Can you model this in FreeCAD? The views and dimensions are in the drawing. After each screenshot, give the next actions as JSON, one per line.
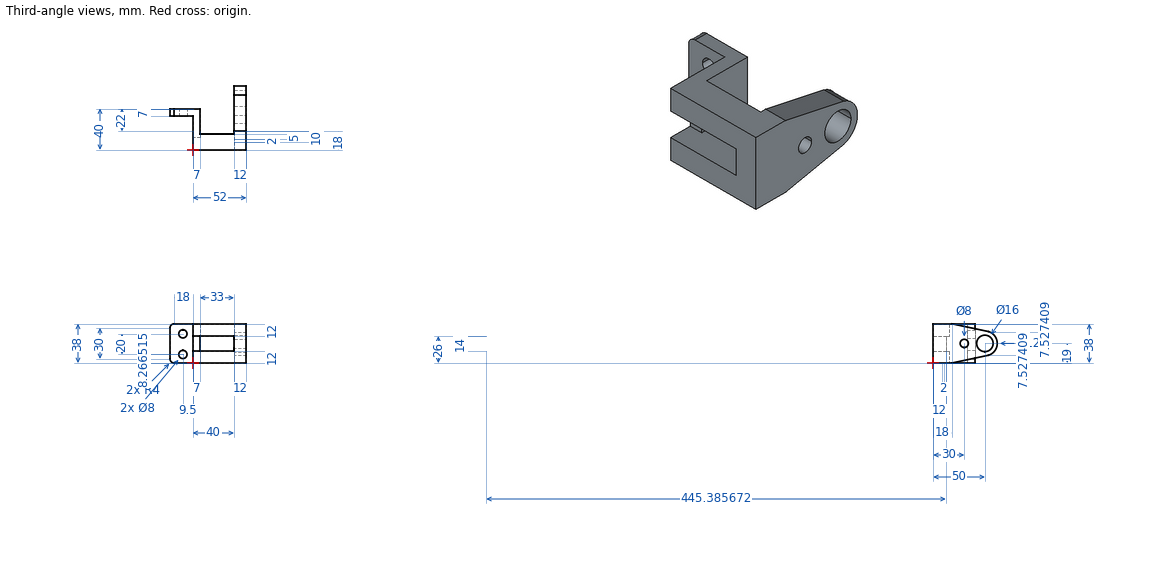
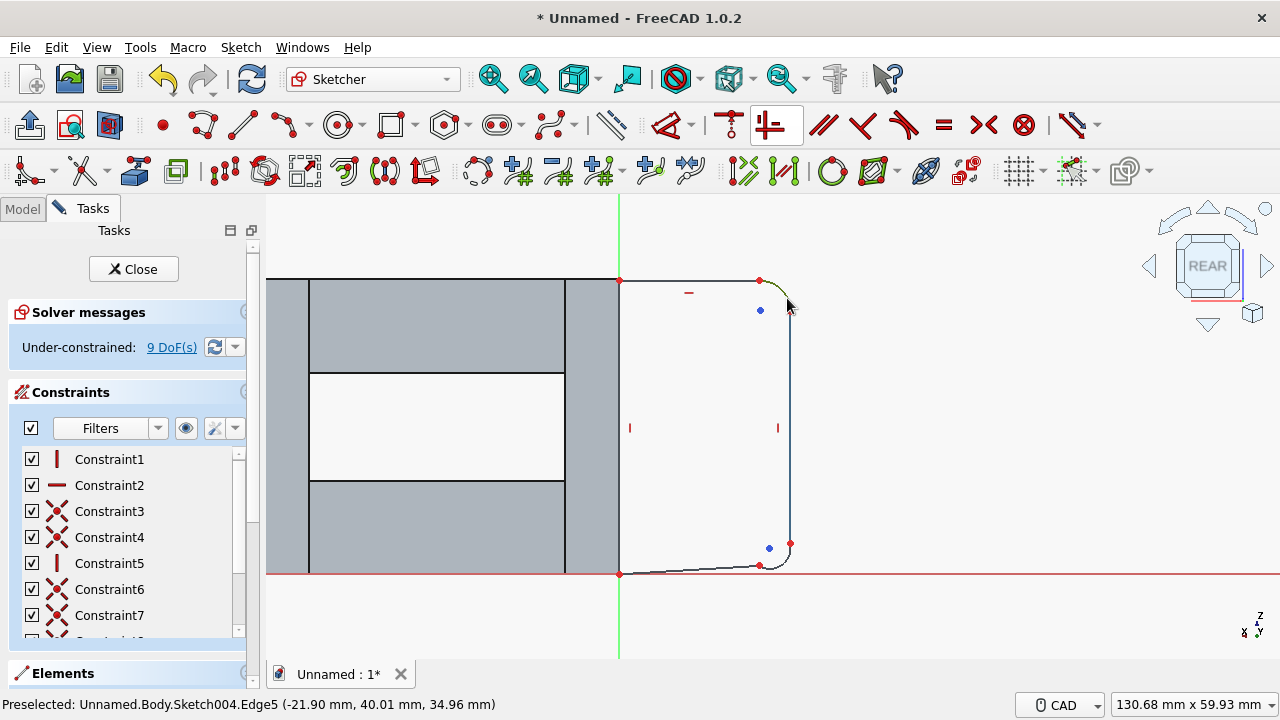
{"action": "left_click", "coordinate": [904, 126]}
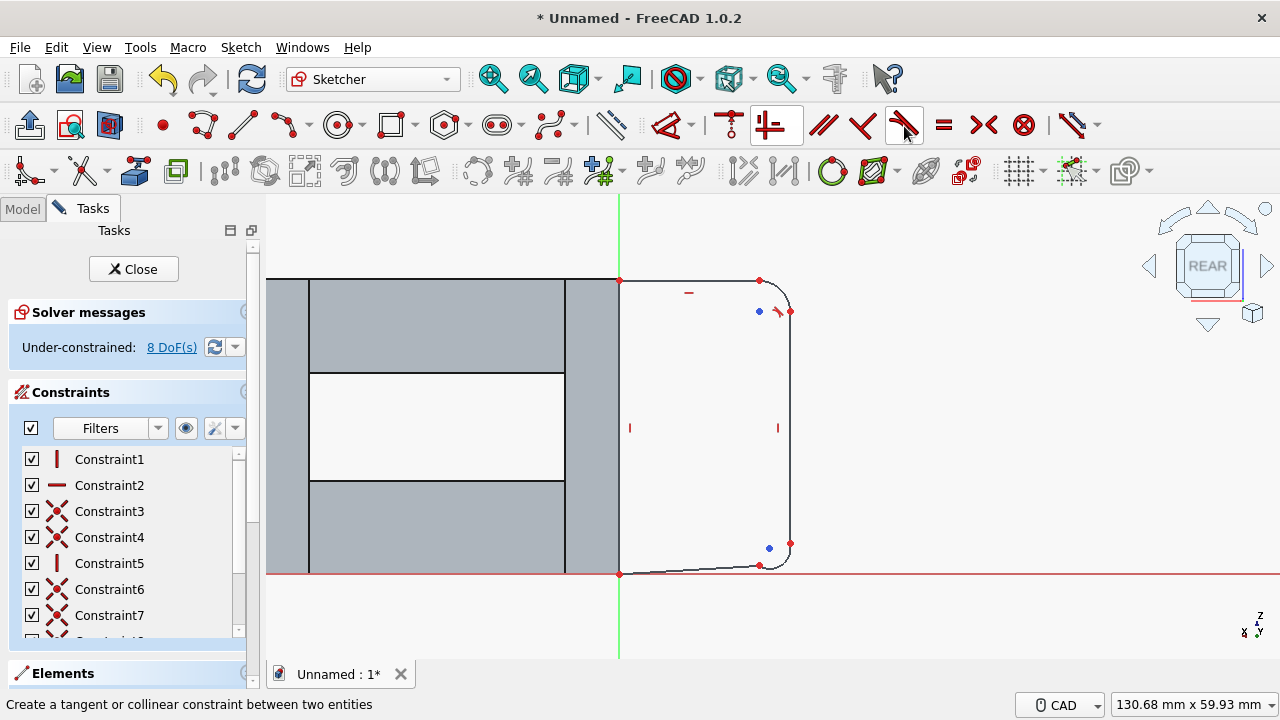
{"action": "left_click", "coordinate": [790, 474]}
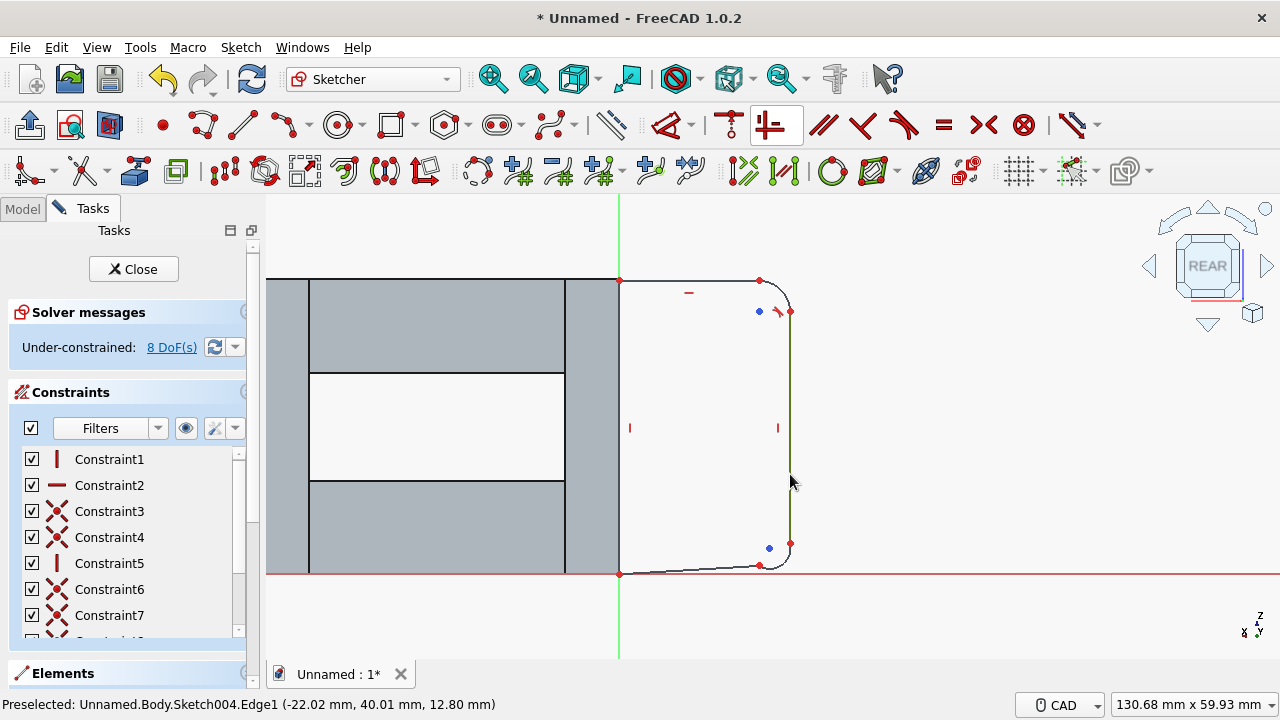
{"action": "left_click", "coordinate": [788, 558]}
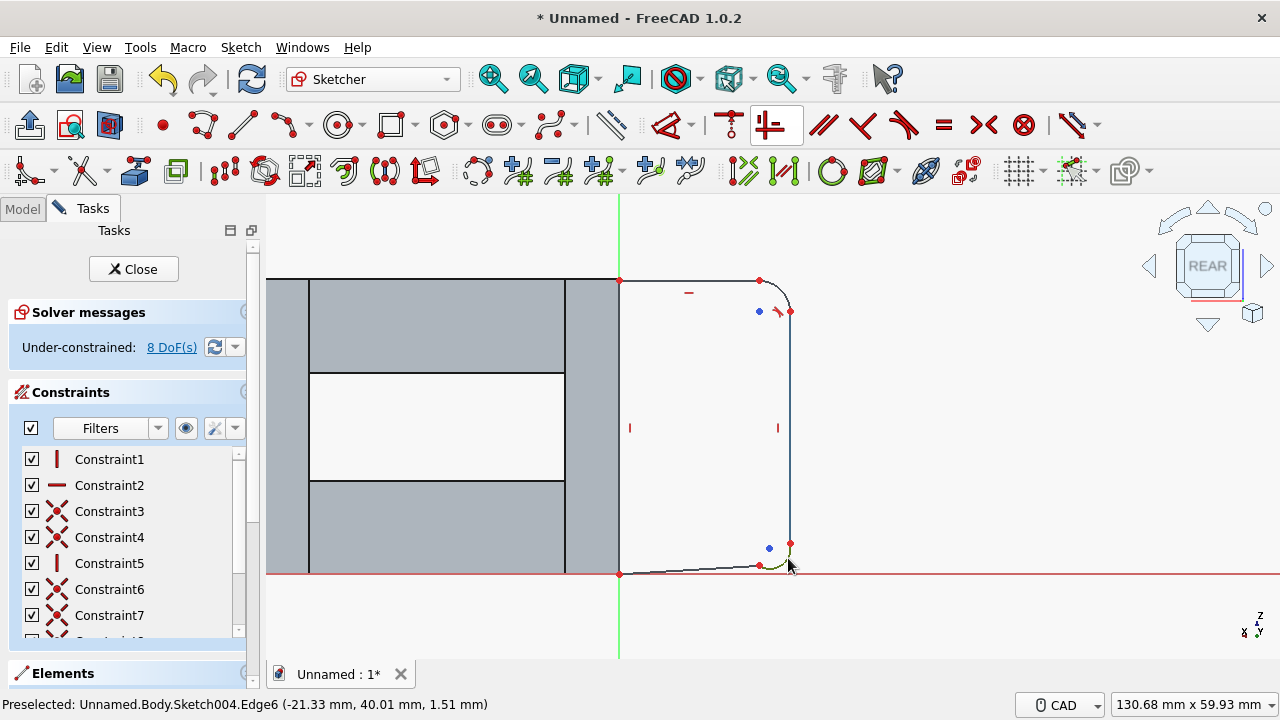
{"action": "left_click", "coordinate": [904, 126]}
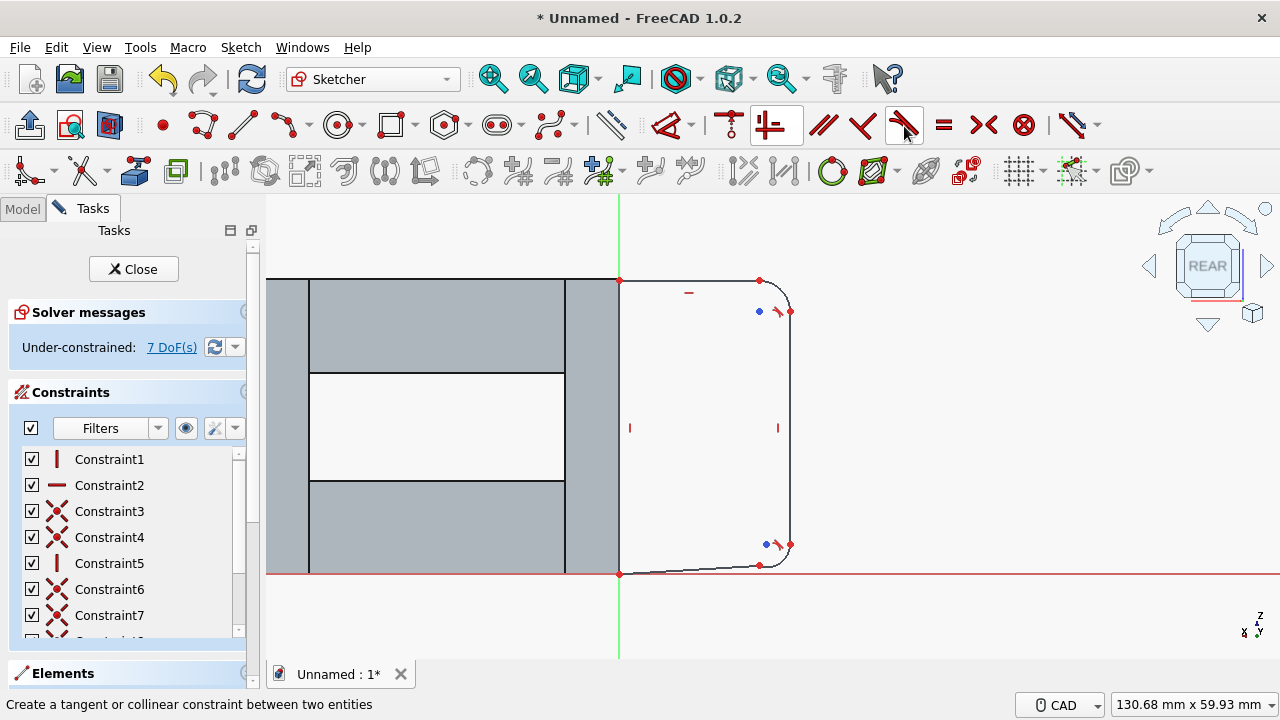
{"action": "left_click", "coordinate": [717, 281]}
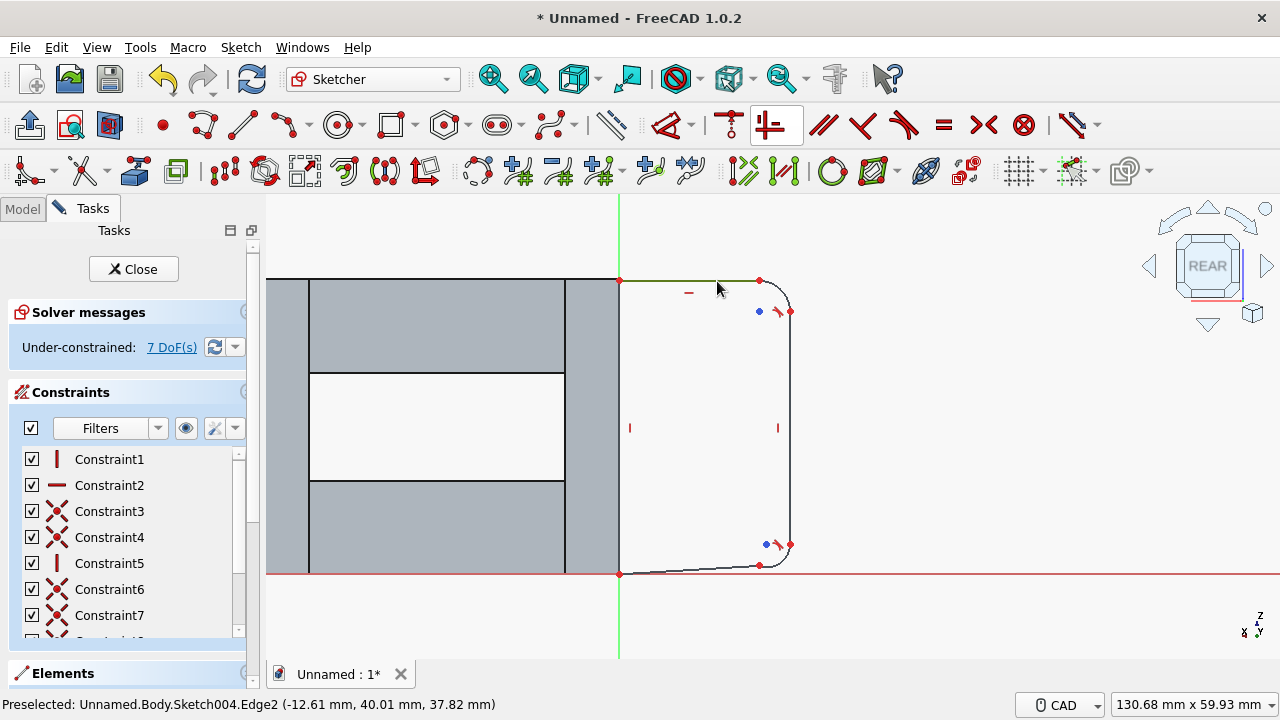
{"action": "left_click", "coordinate": [787, 298]}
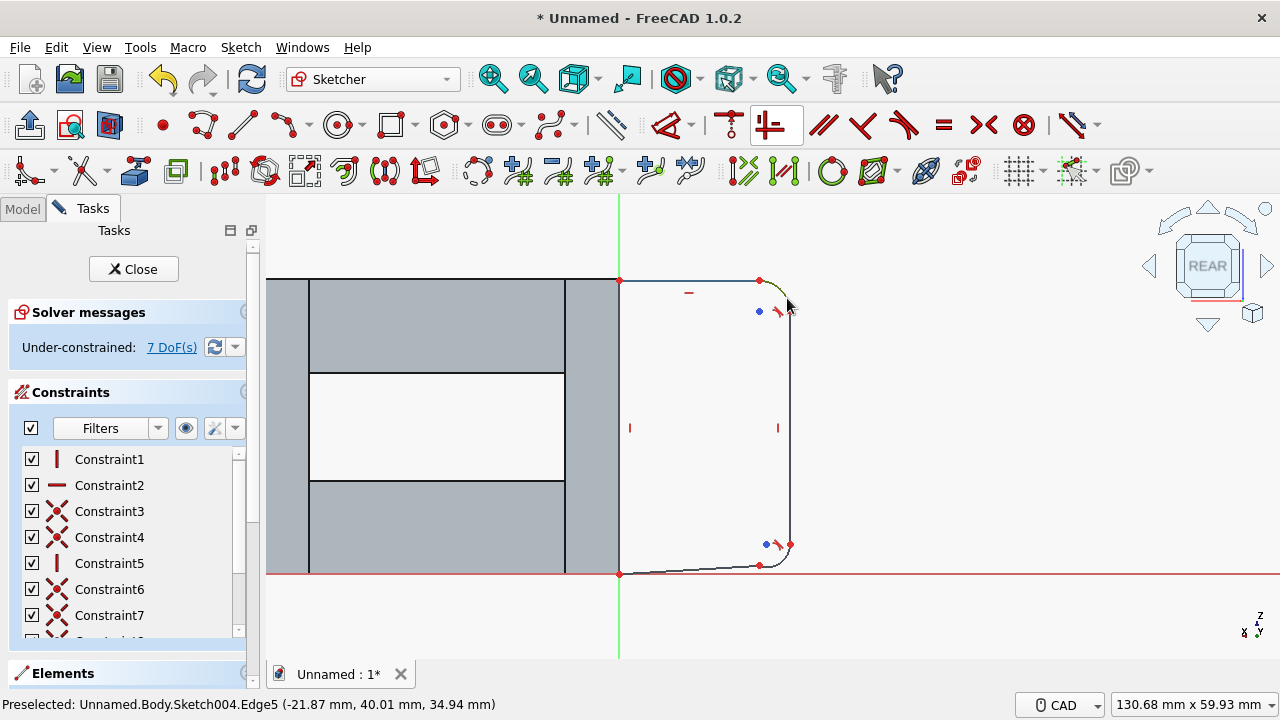
{"action": "left_click", "coordinate": [904, 126]}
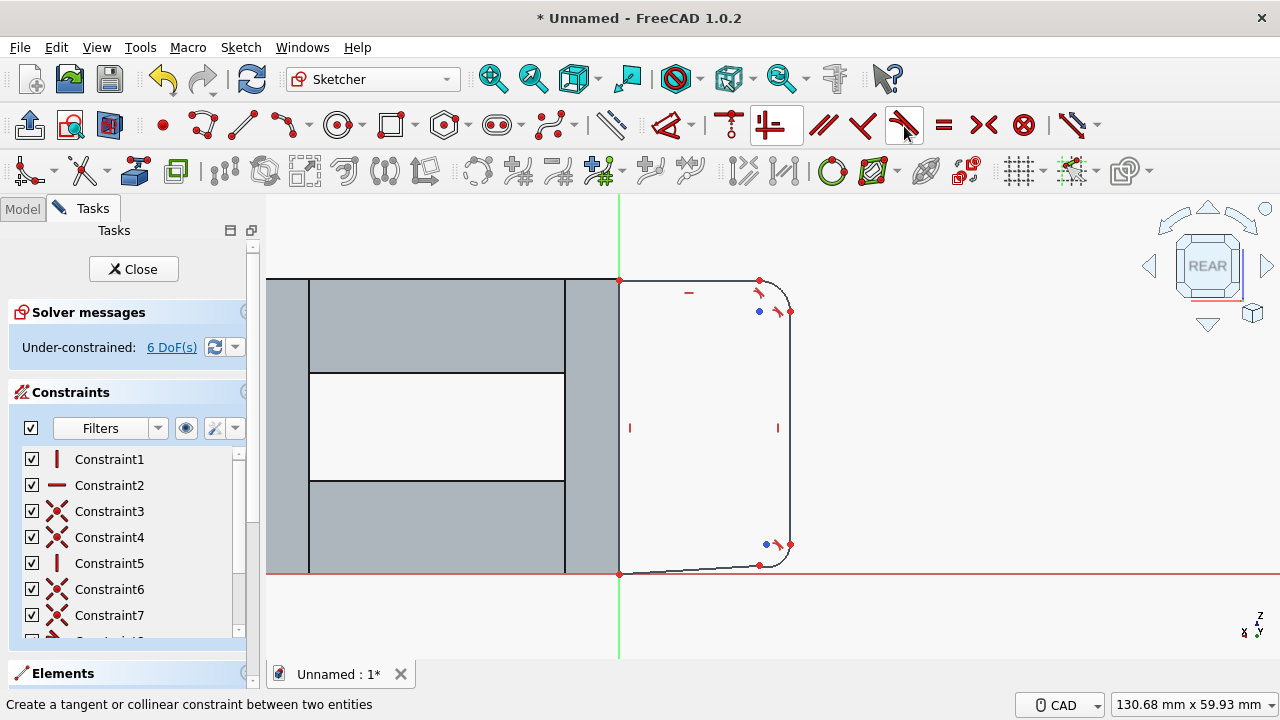
{"action": "left_click", "coordinate": [661, 572]}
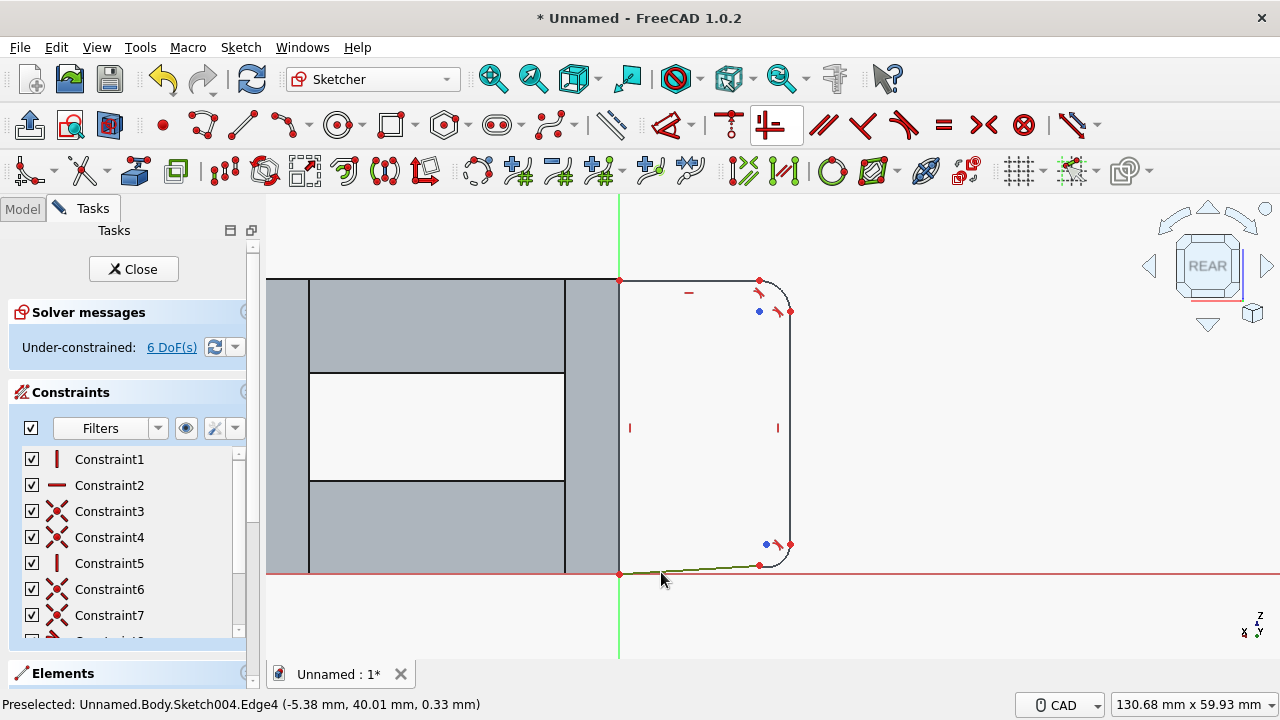
{"action": "left_click", "coordinate": [786, 557]}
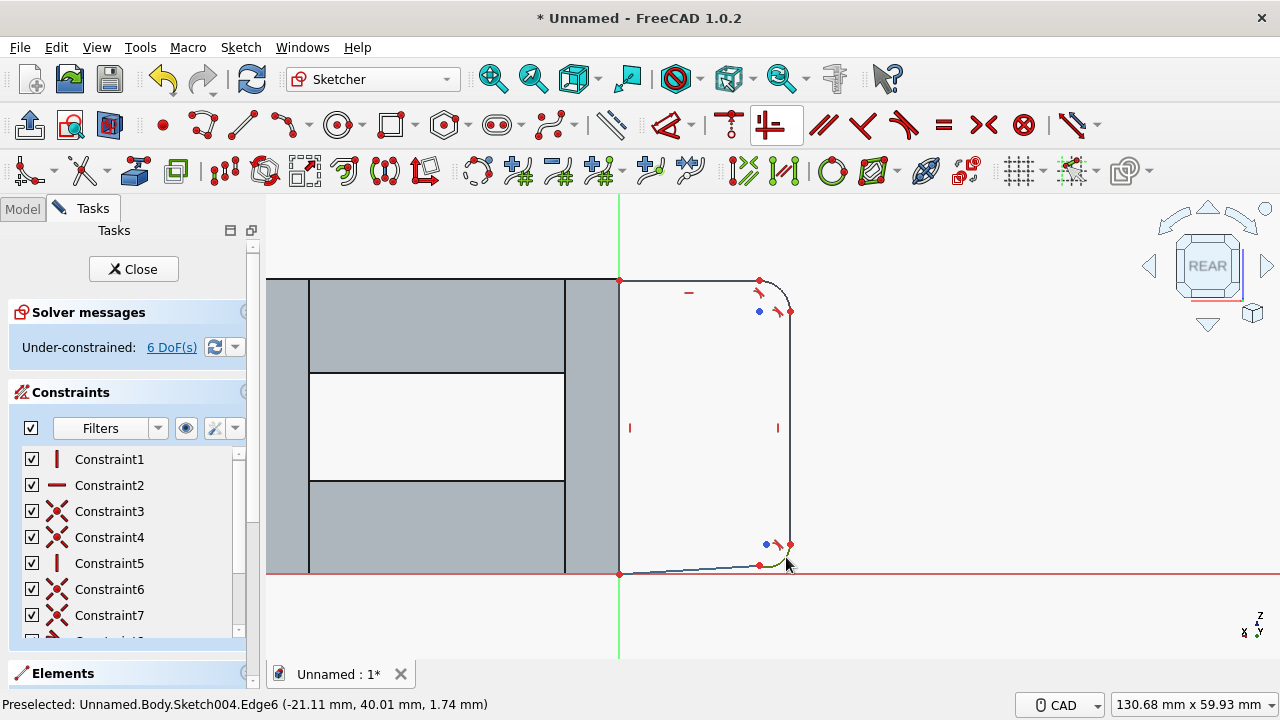
{"action": "left_click", "coordinate": [904, 126]}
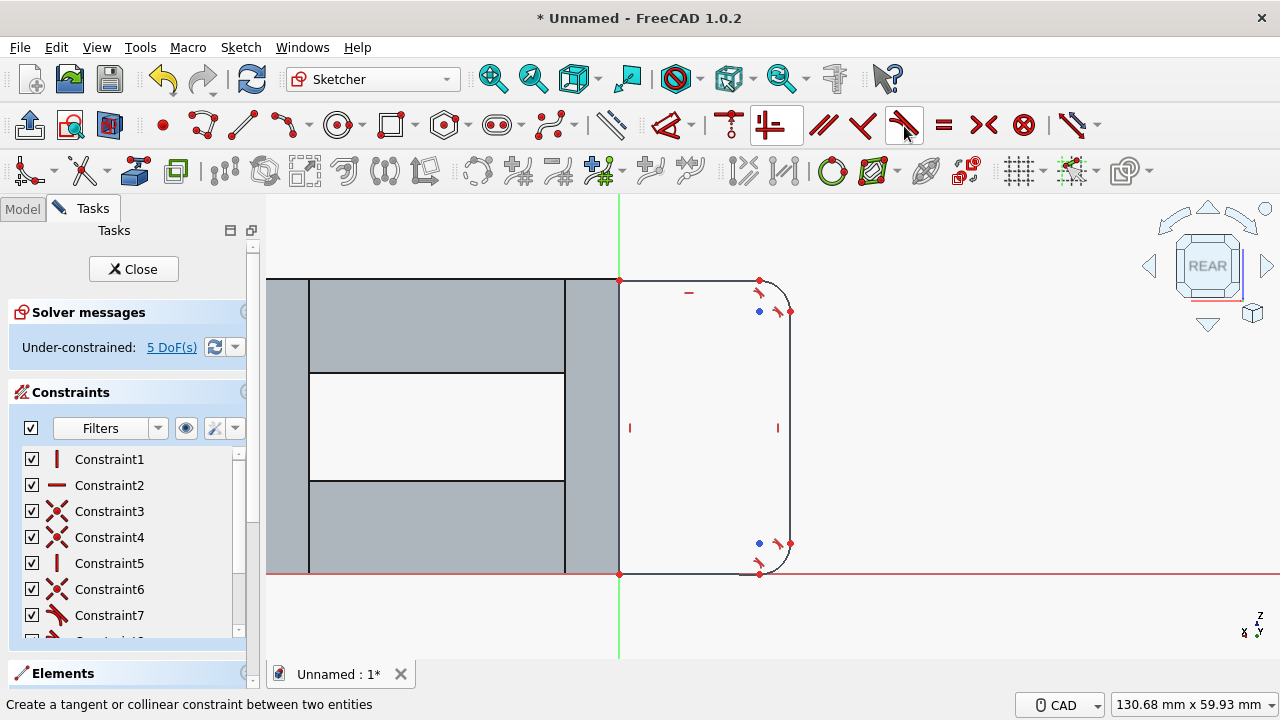
{"action": "left_click", "coordinate": [661, 574]}